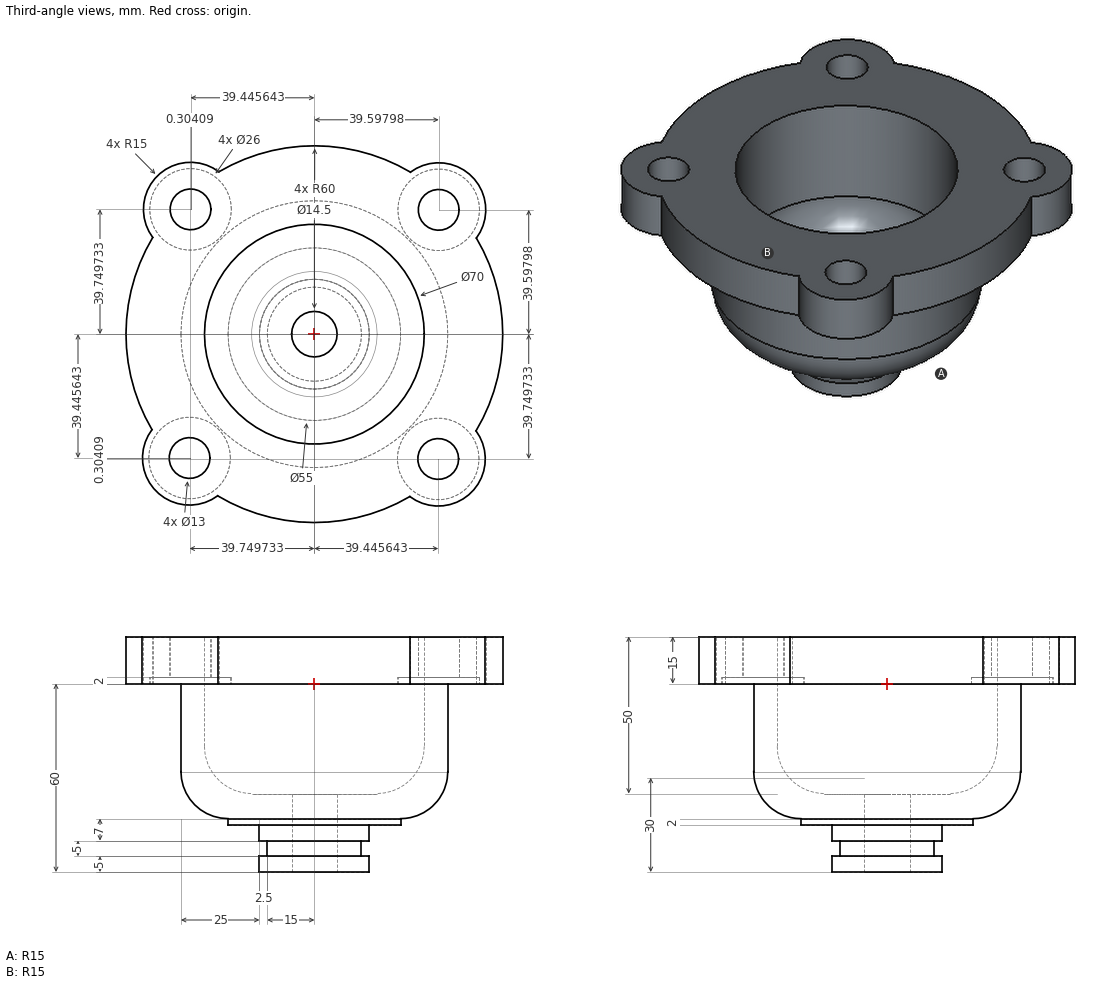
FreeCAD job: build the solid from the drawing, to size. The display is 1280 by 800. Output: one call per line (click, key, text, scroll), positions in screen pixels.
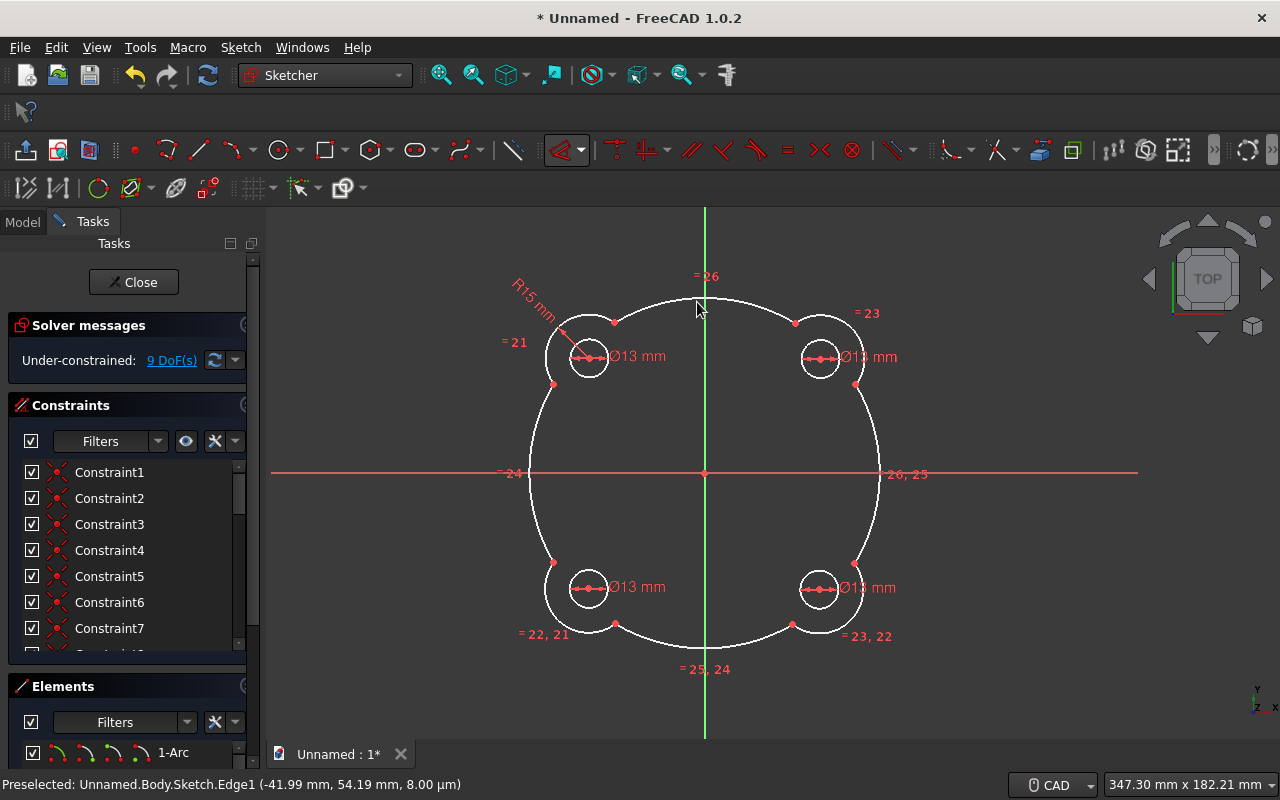
click(533, 436)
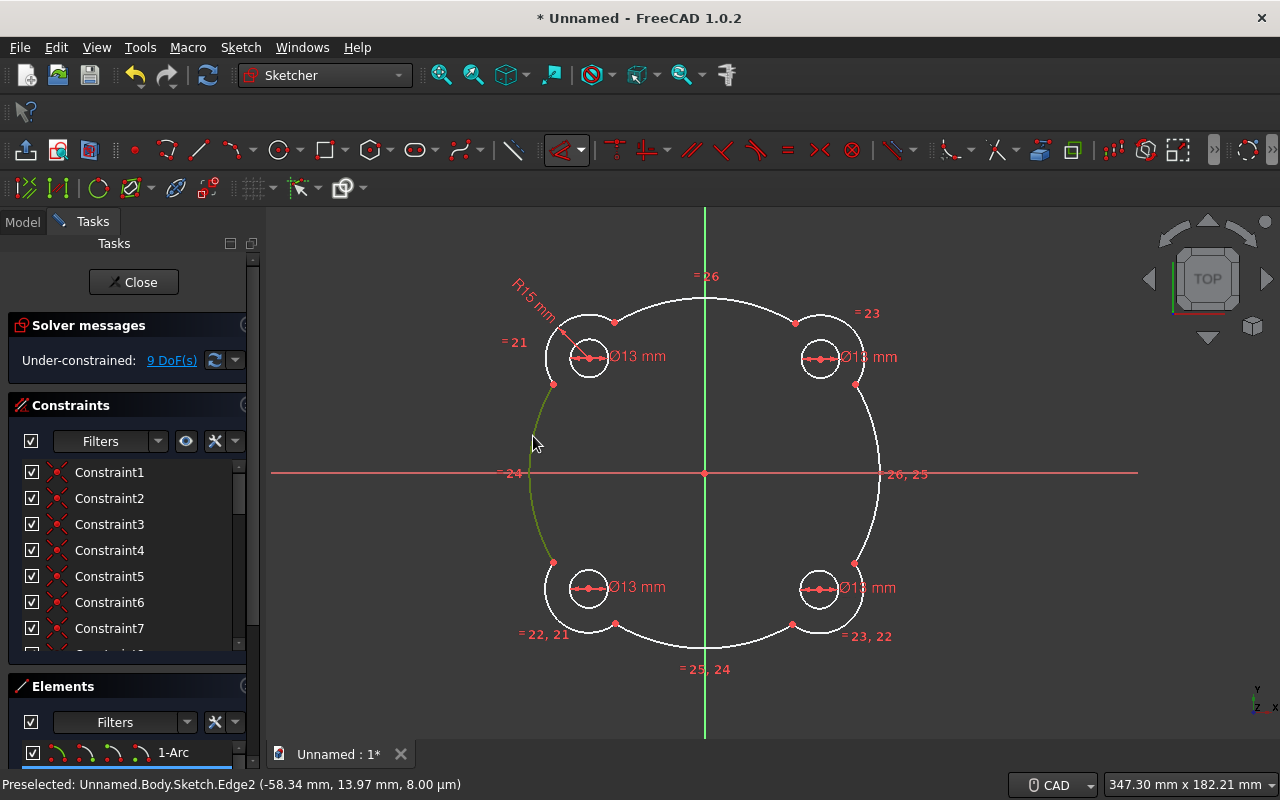
key(k)
key(r)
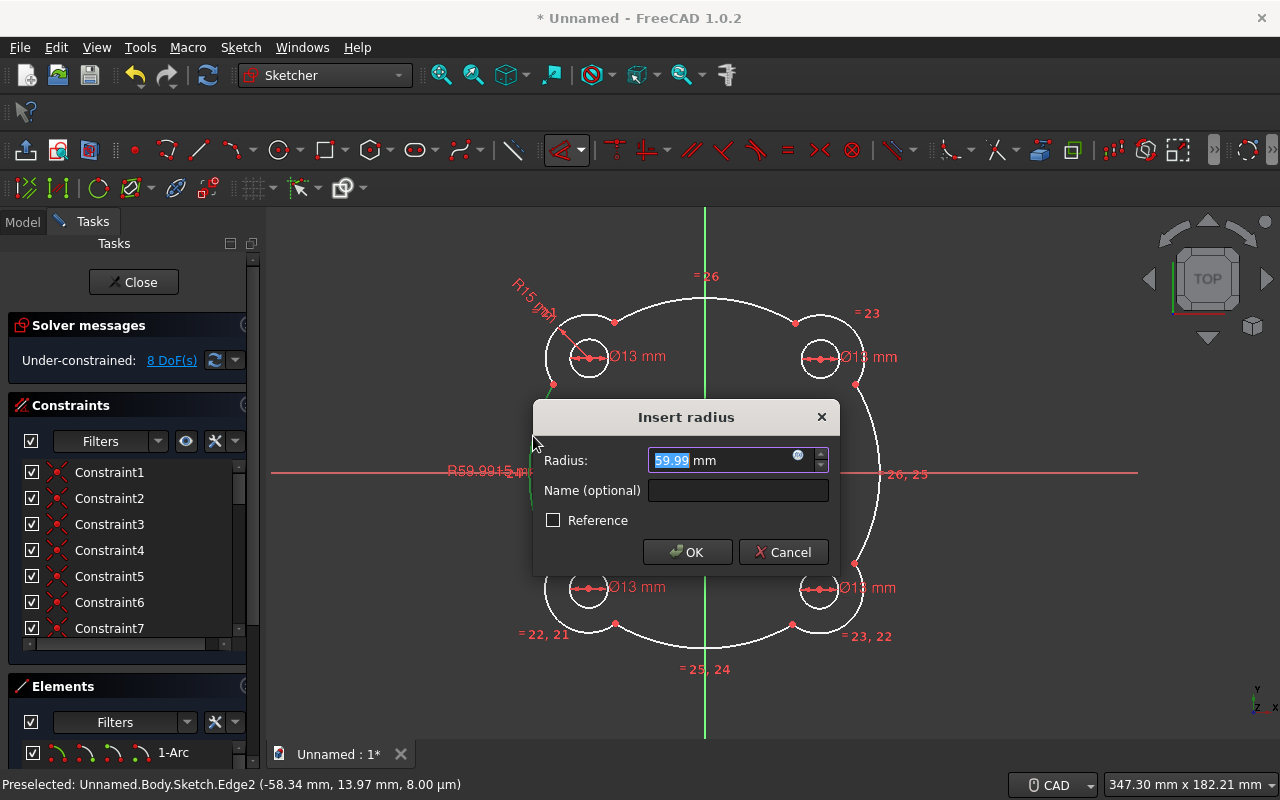
text(60)
key(Return)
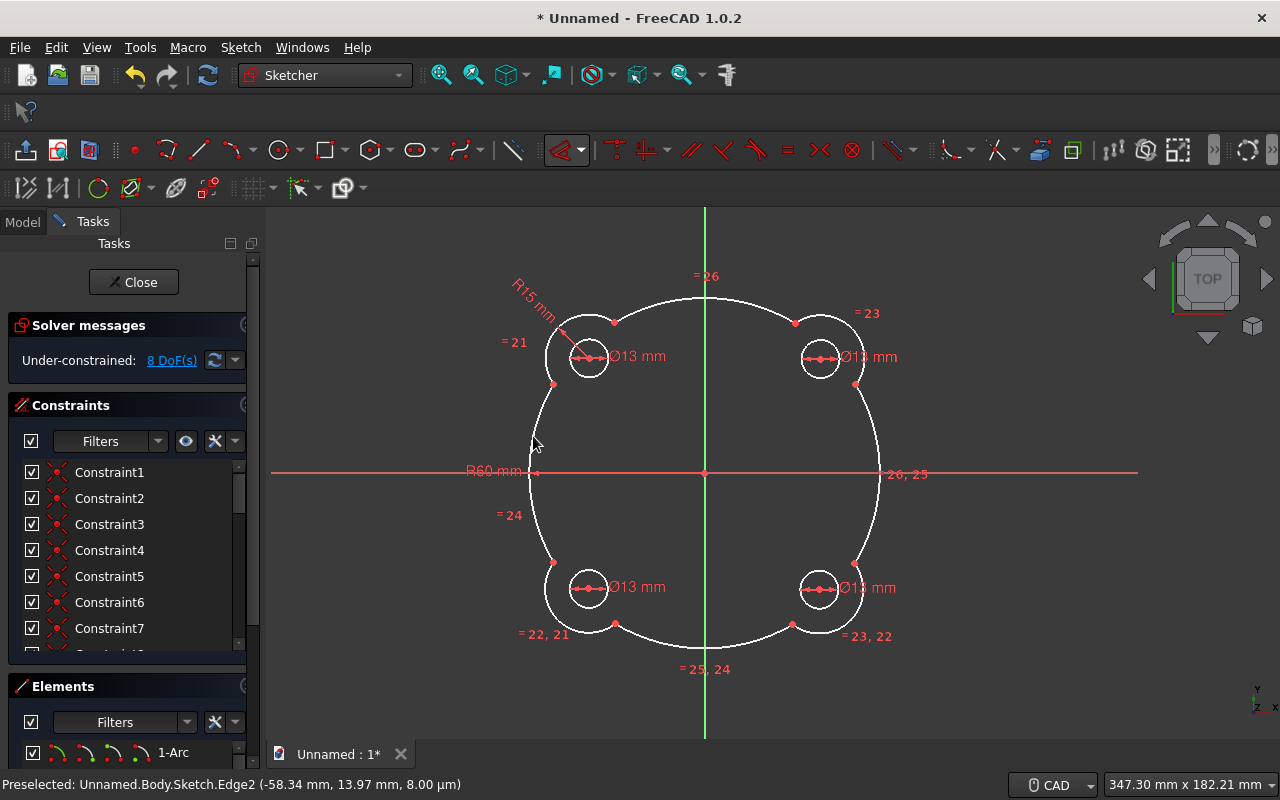
click(821, 359)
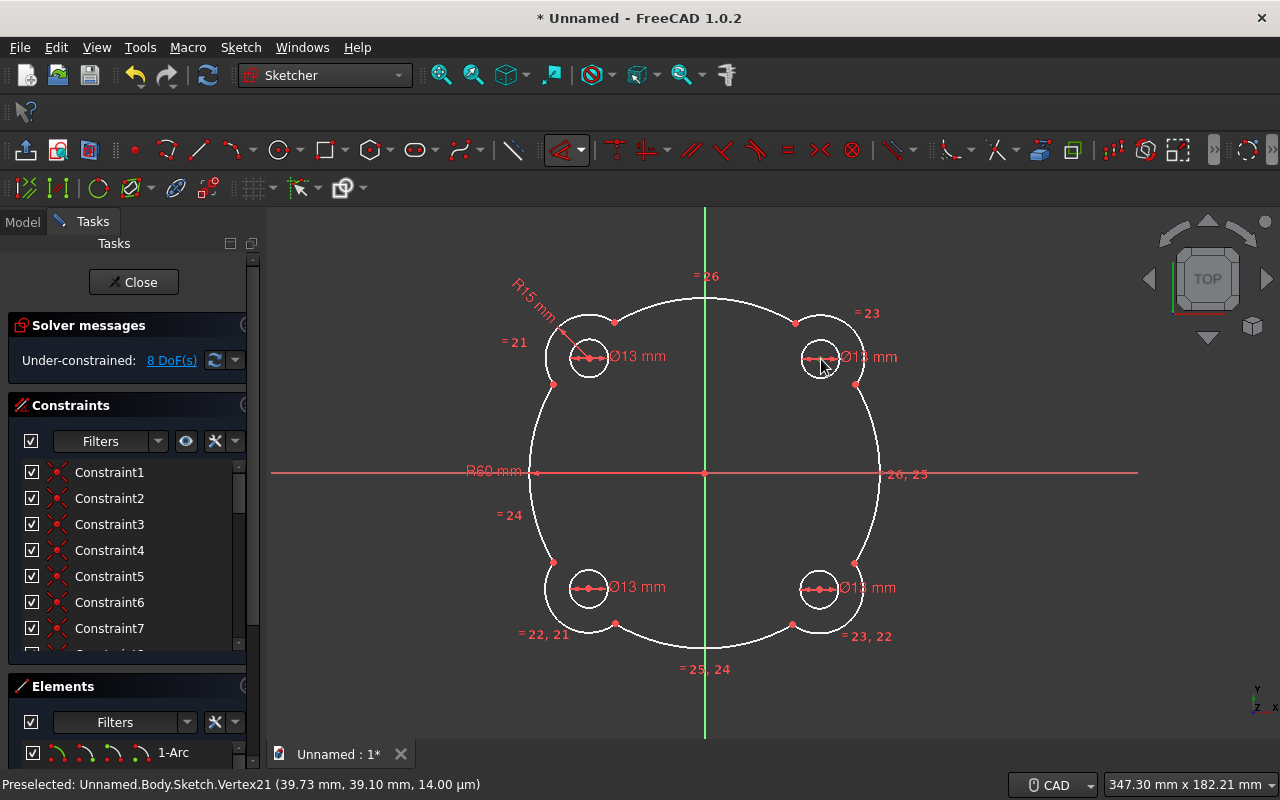
click(584, 150)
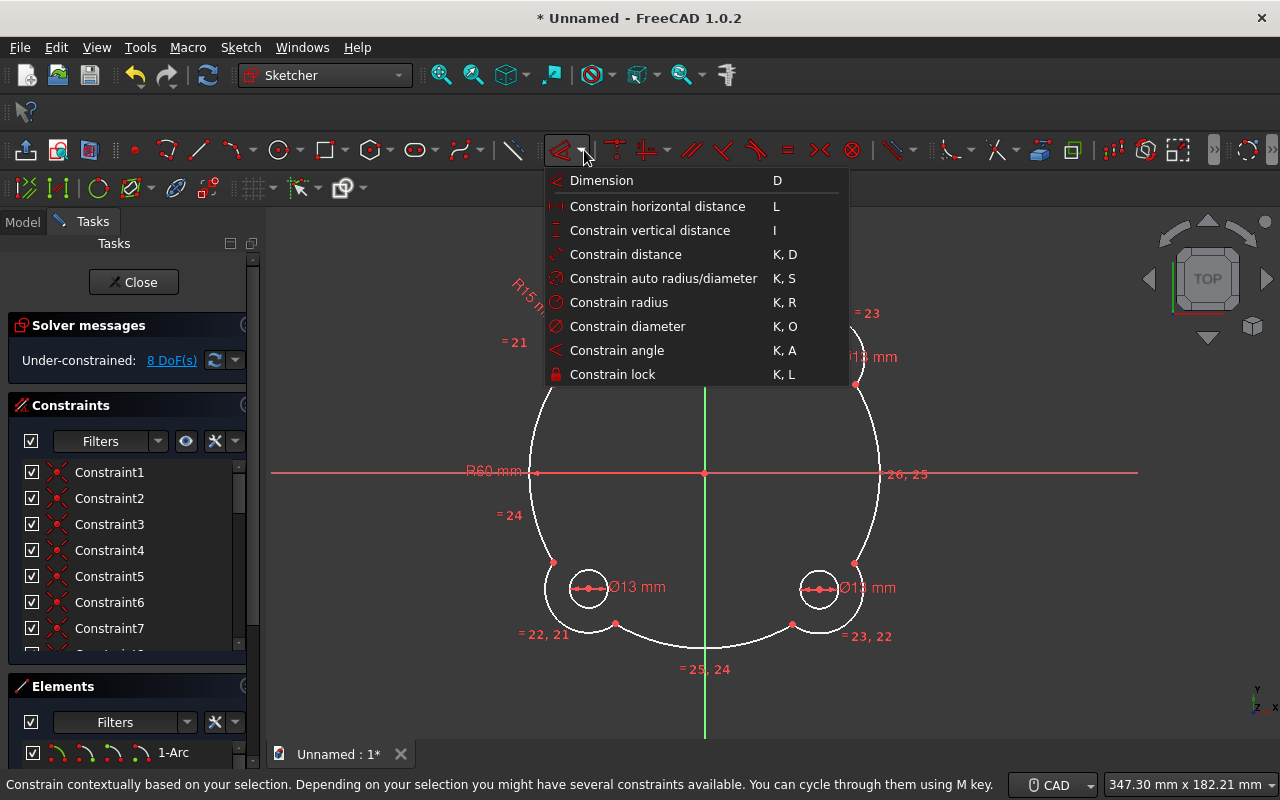
click(697, 206)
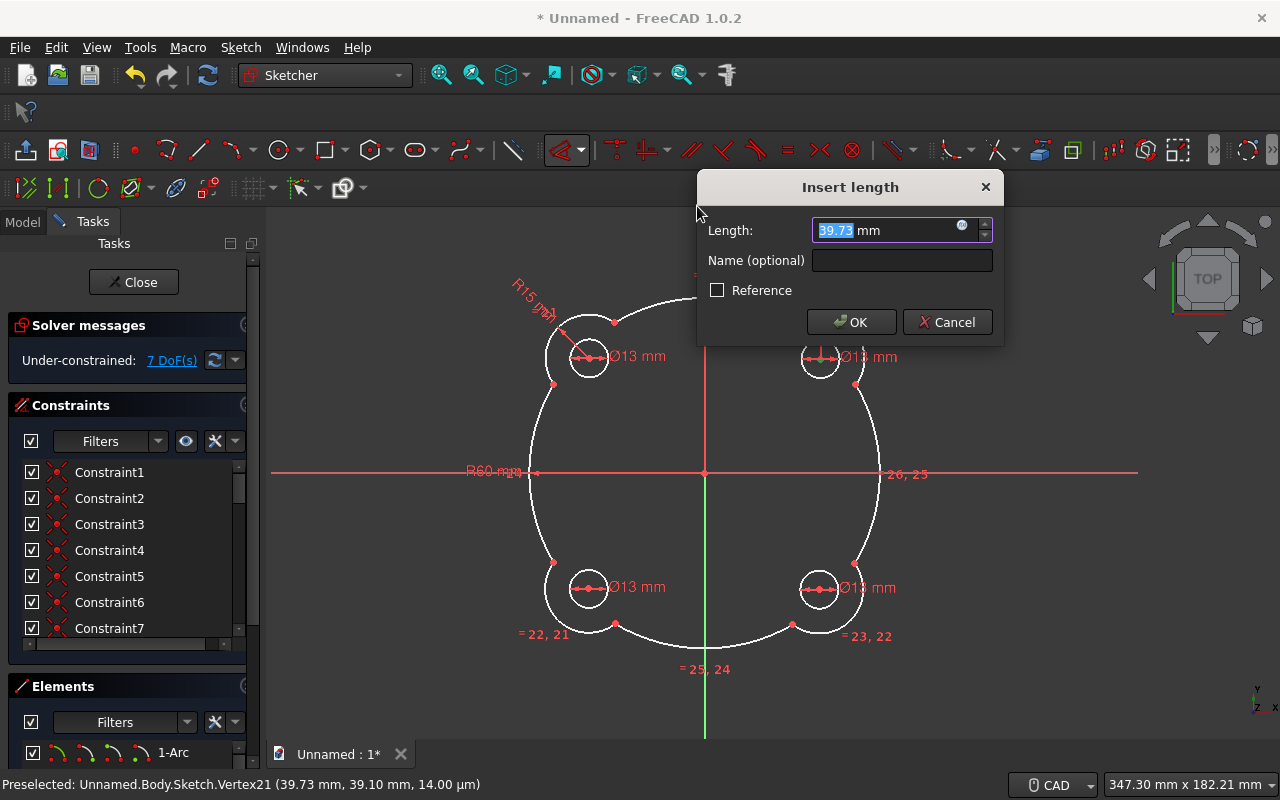
text(39.59798)
key(Return)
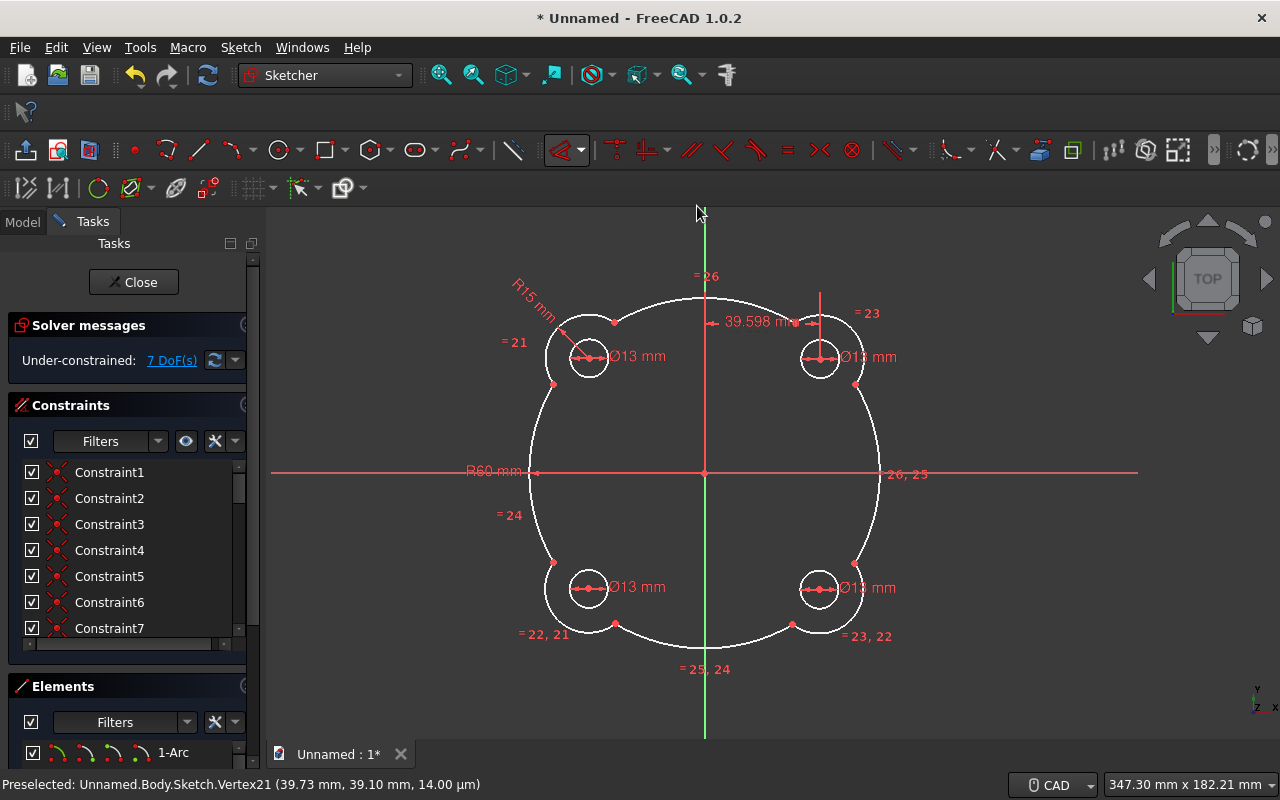
click(820, 359)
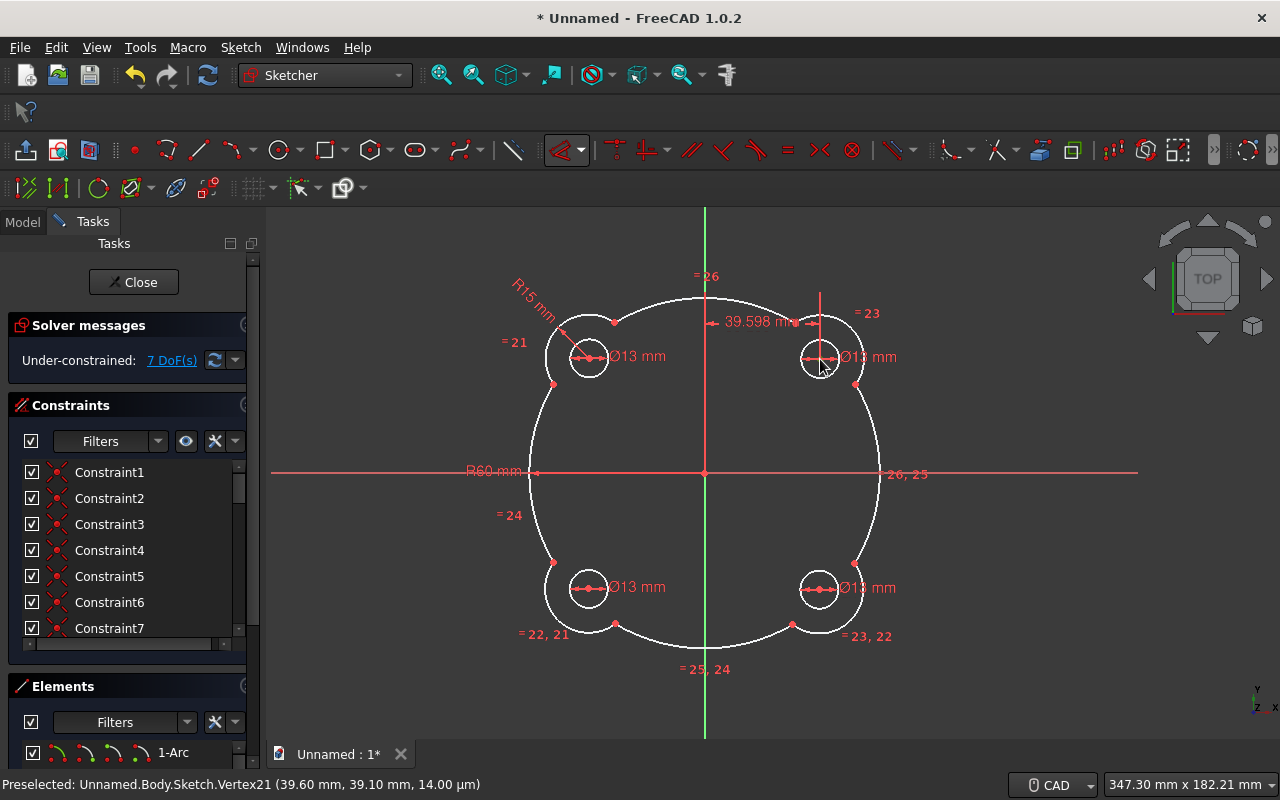
click(584, 150)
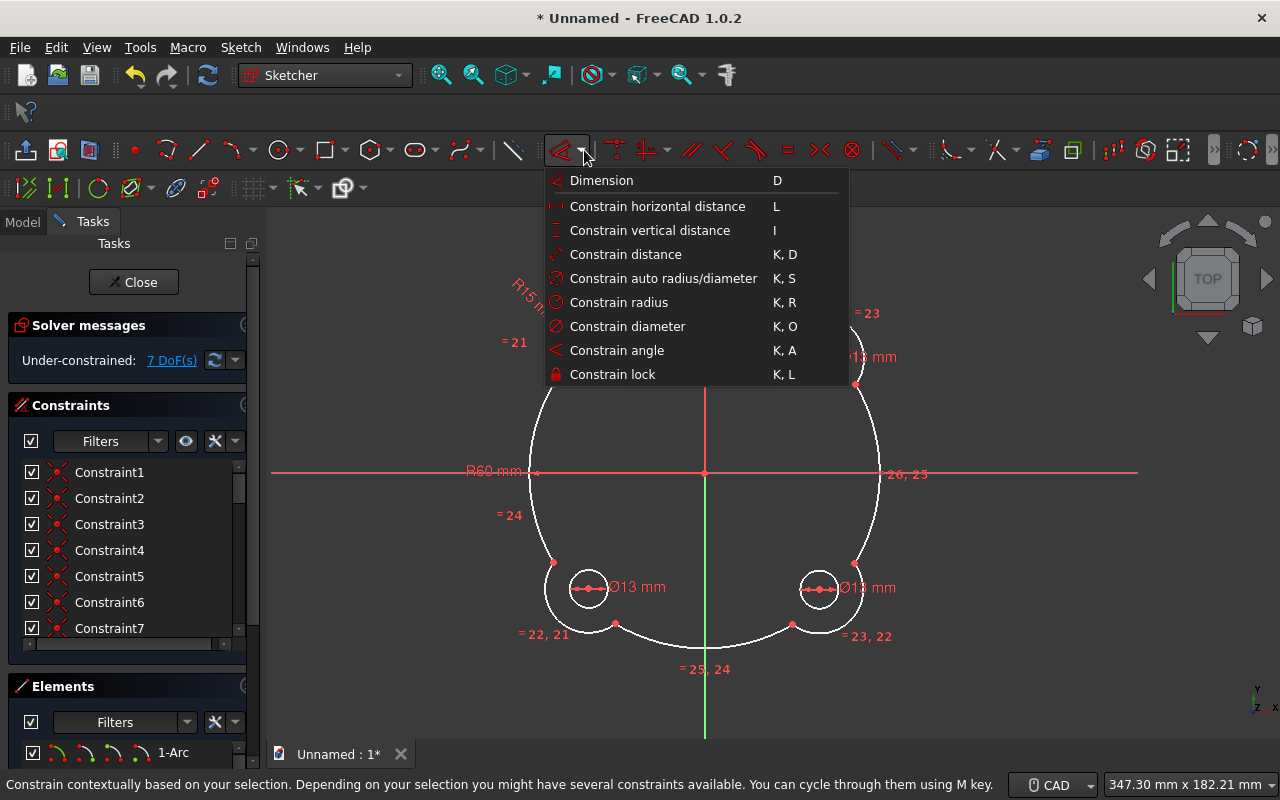
click(697, 230)